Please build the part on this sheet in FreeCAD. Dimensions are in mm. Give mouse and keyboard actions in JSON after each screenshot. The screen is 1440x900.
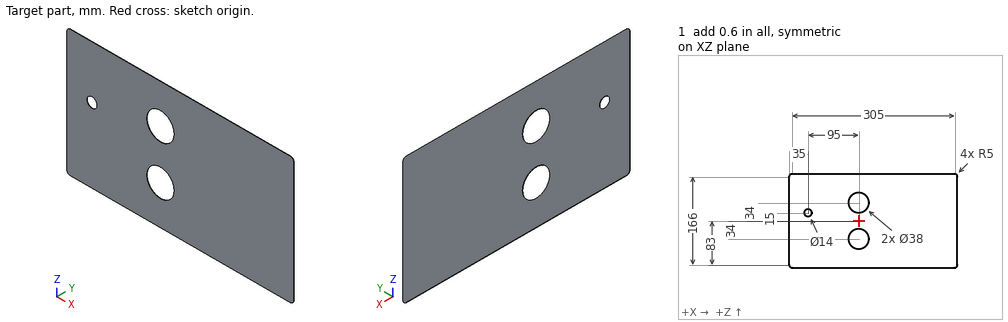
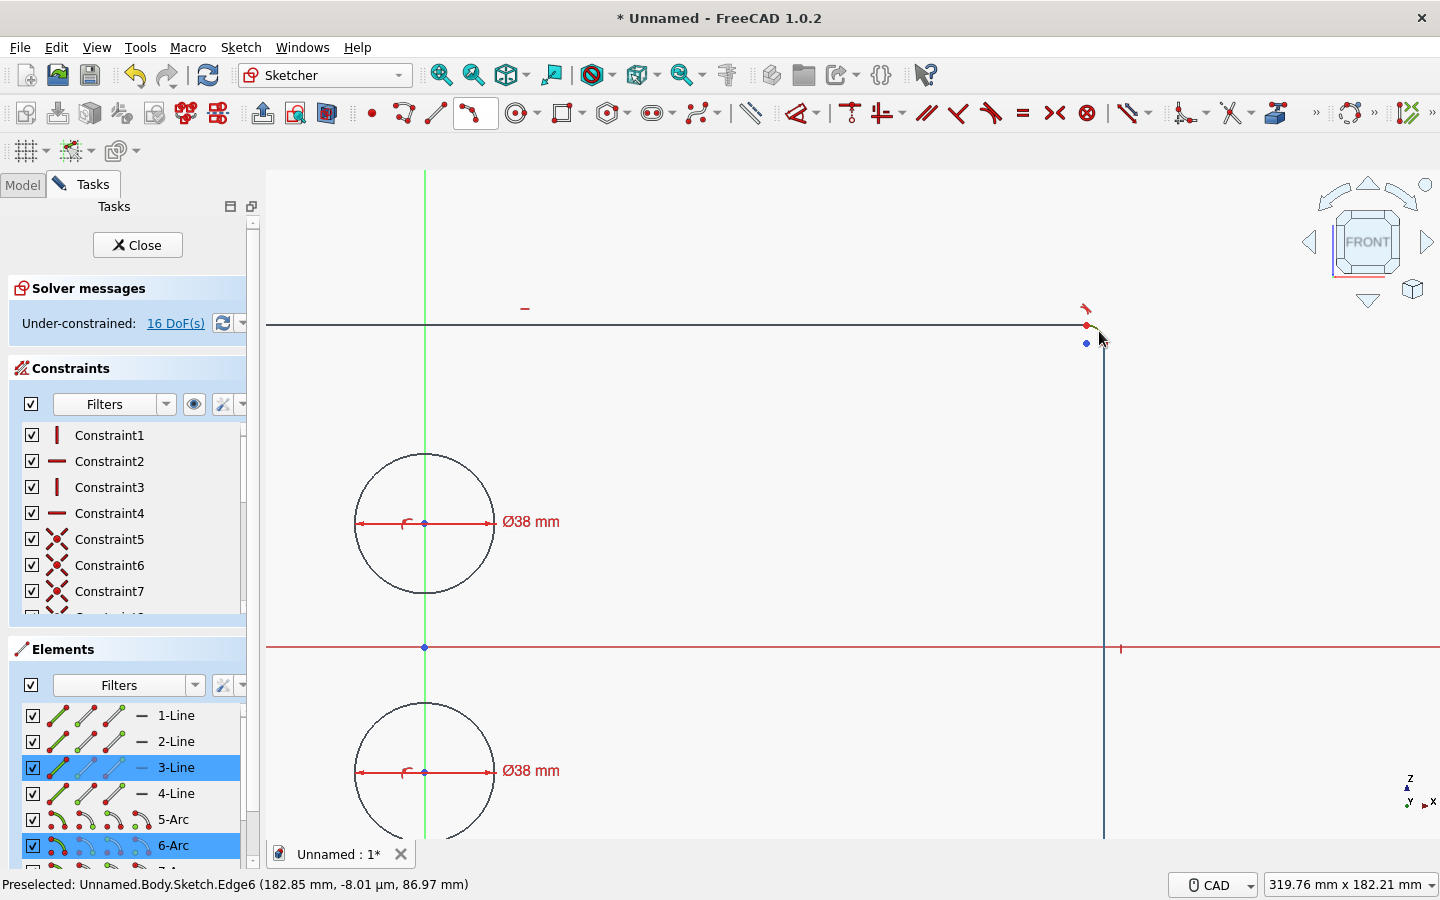
{"action": "left_click", "coordinate": [992, 114]}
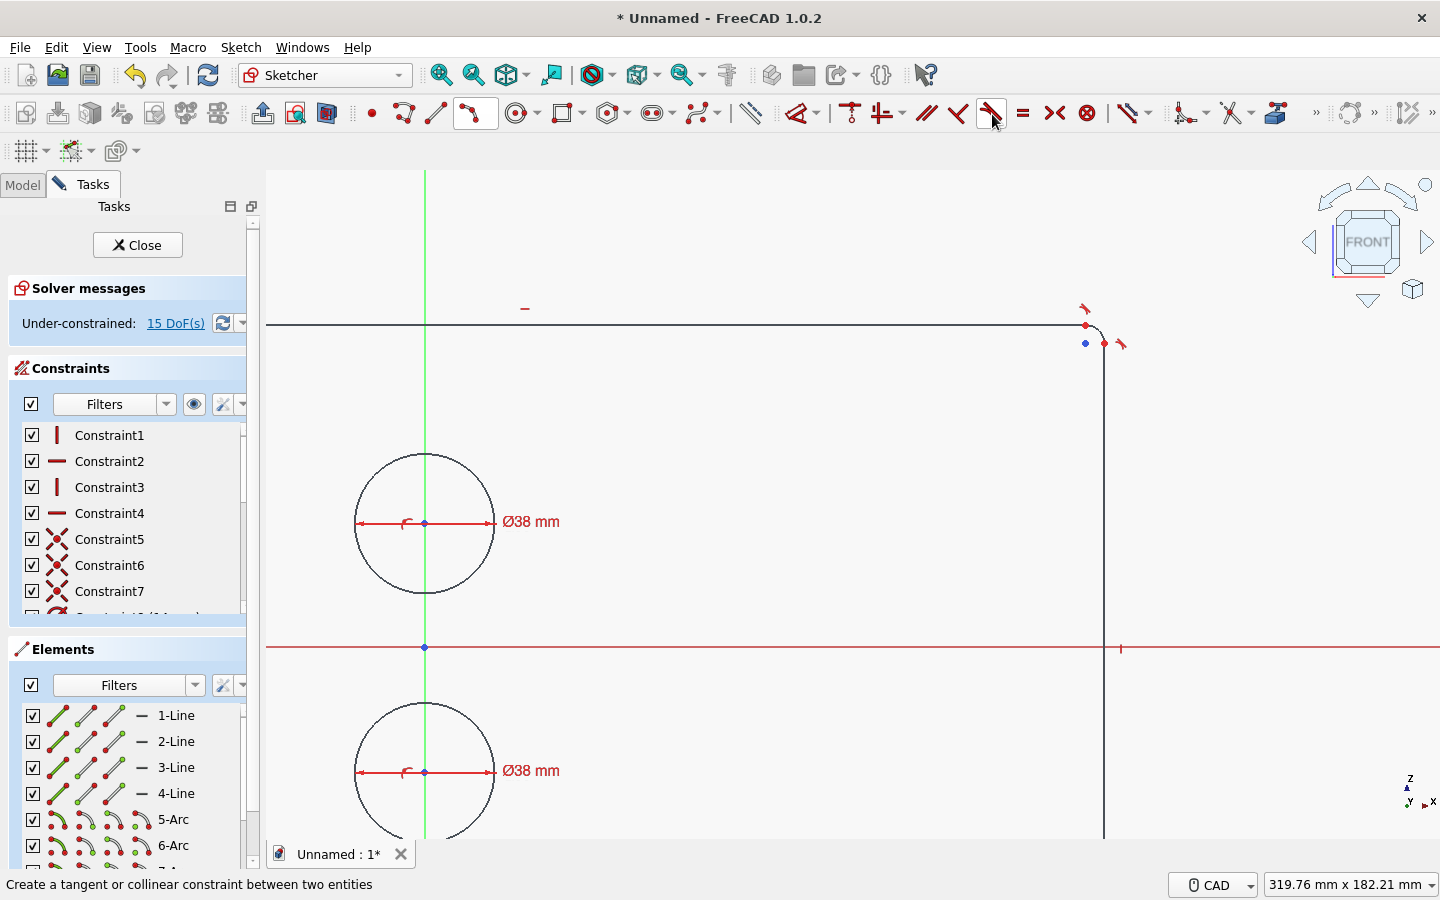
{"action": "left_click", "coordinate": [1104, 527]}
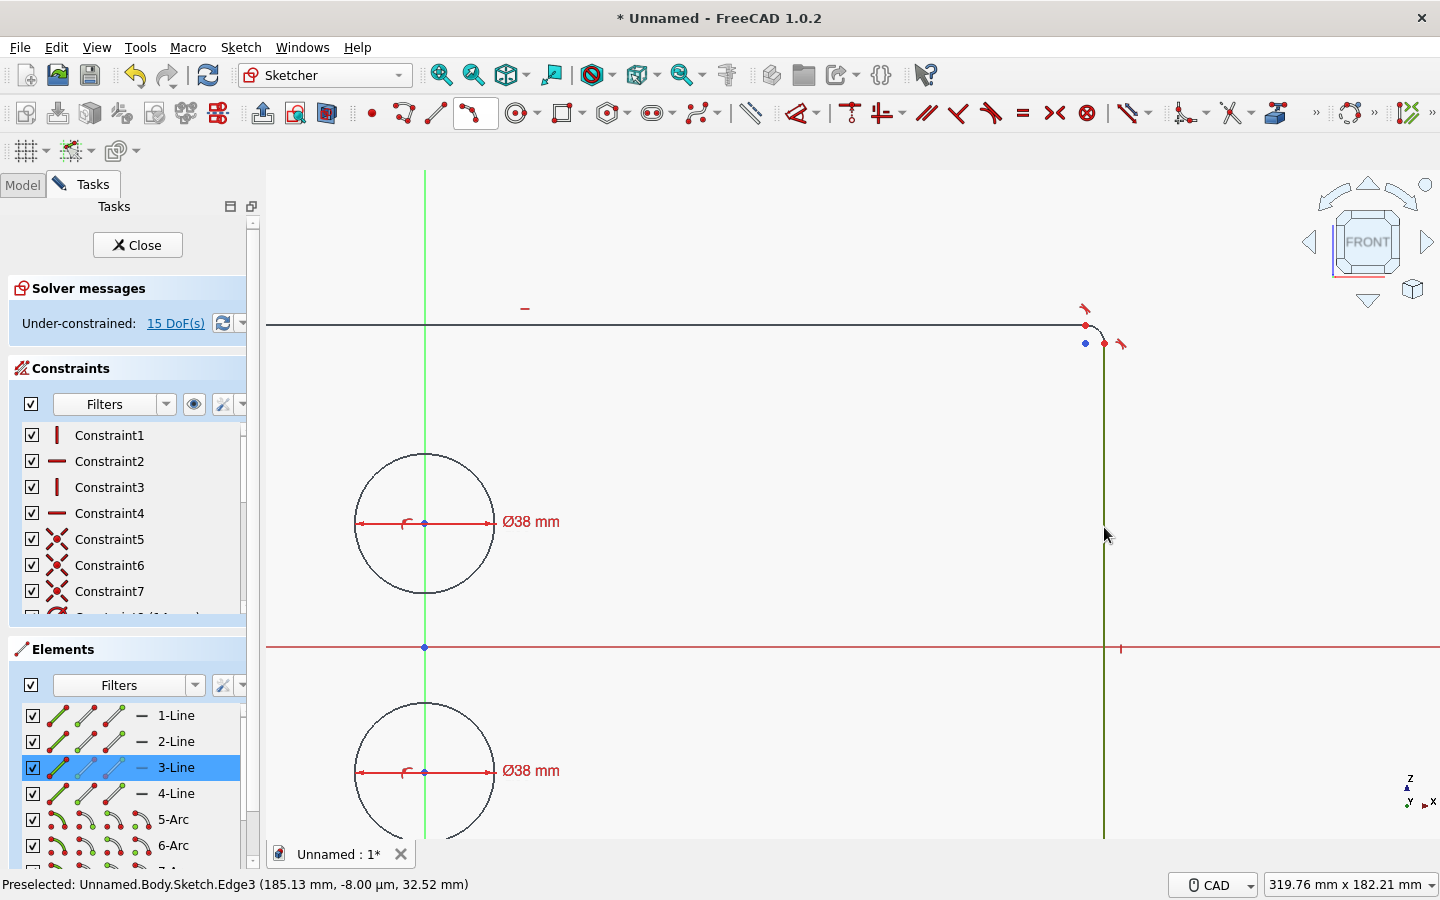
{"action": "scroll", "coordinate": [1099, 331], "scroll_direction": "down", "scroll_amount": 3}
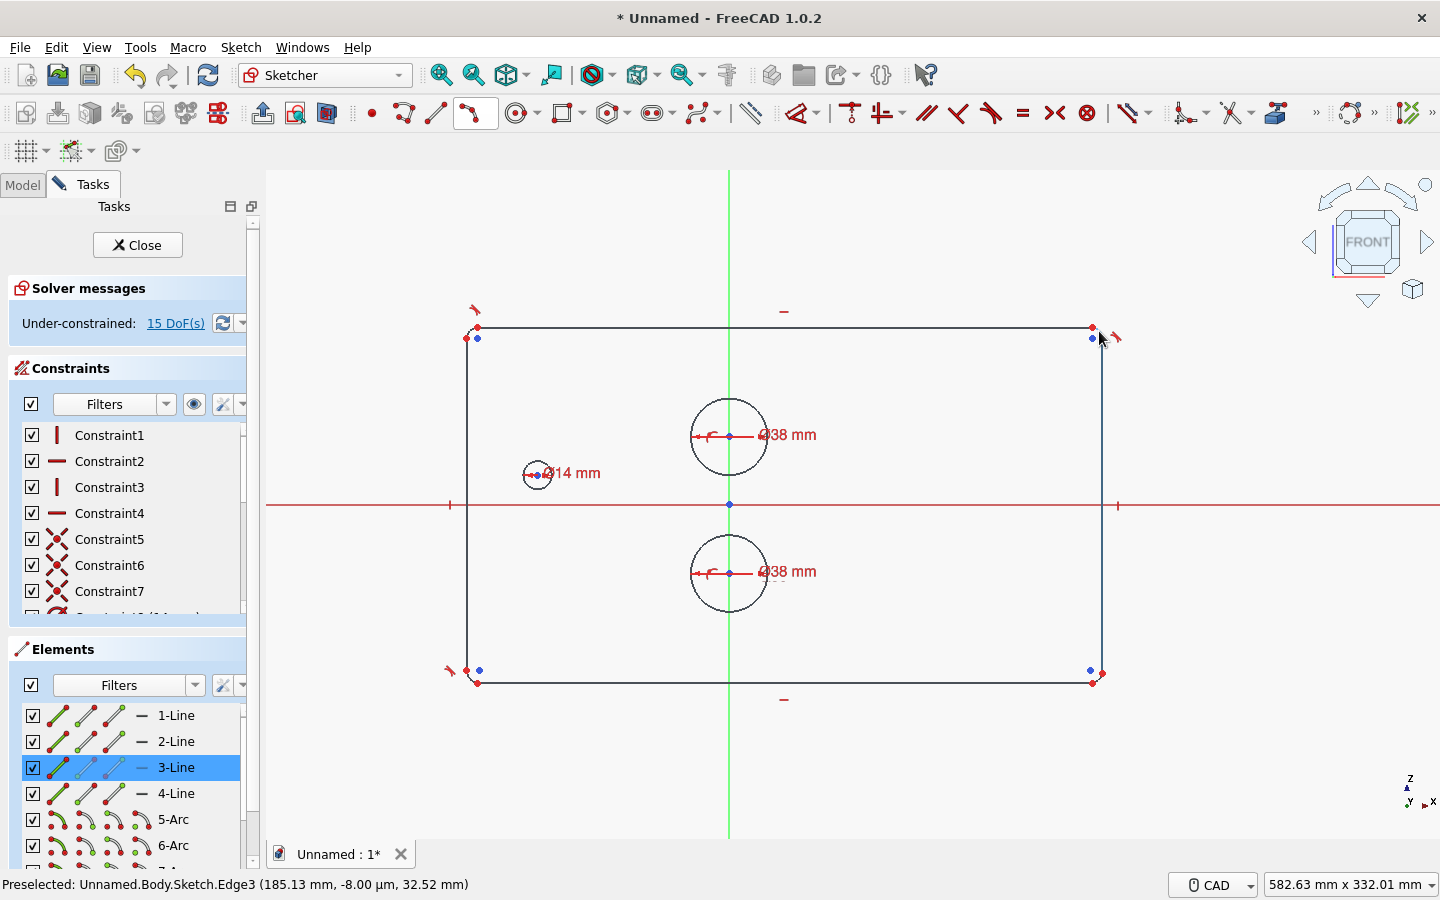
{"action": "scroll", "coordinate": [1099, 680], "scroll_direction": "up", "scroll_amount": 4}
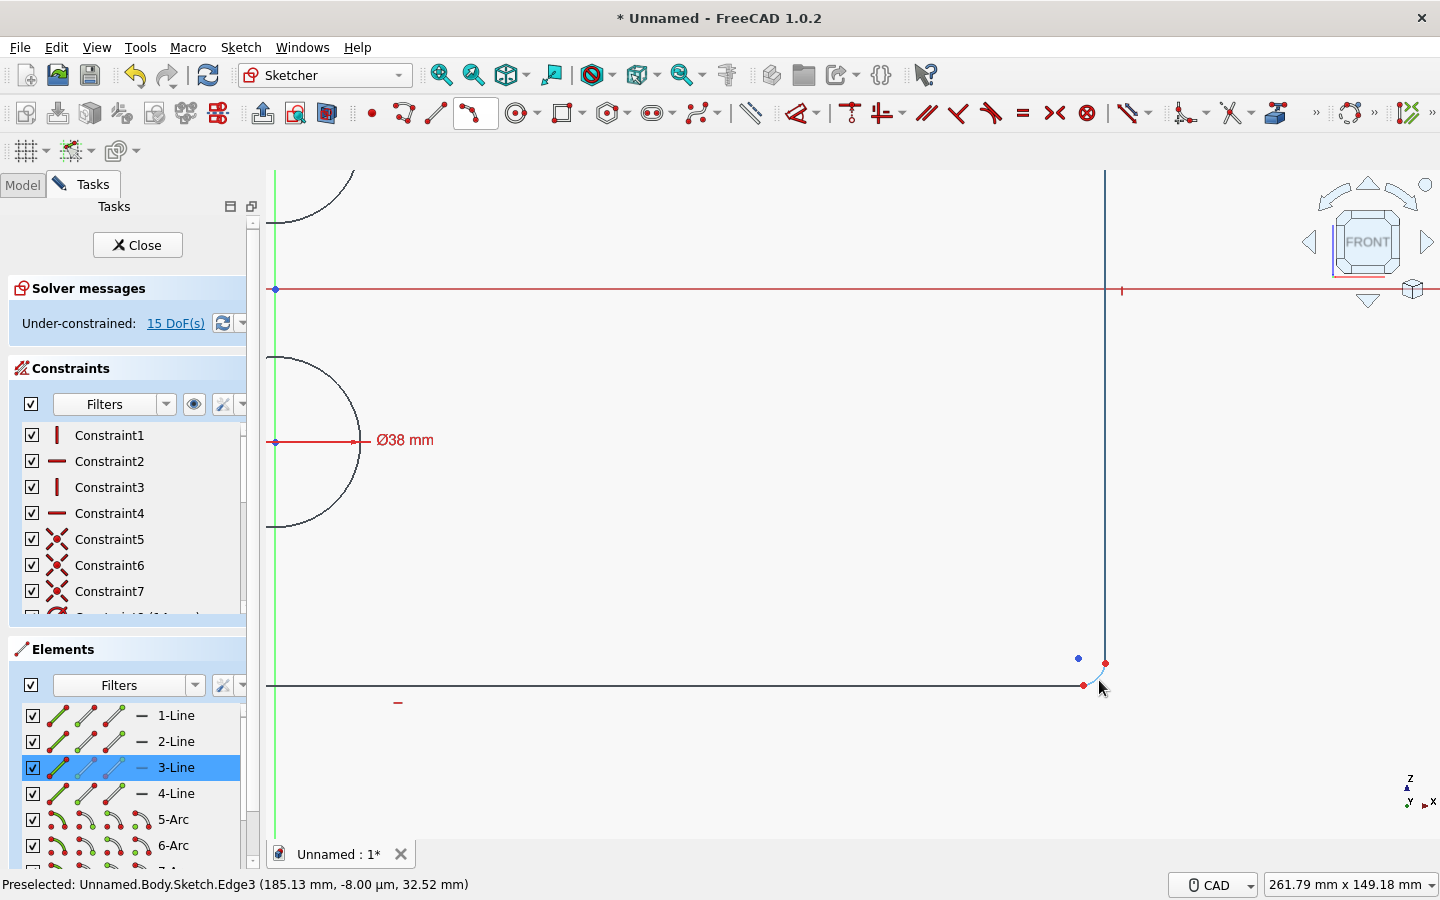
{"action": "left_click", "coordinate": [1098, 678]}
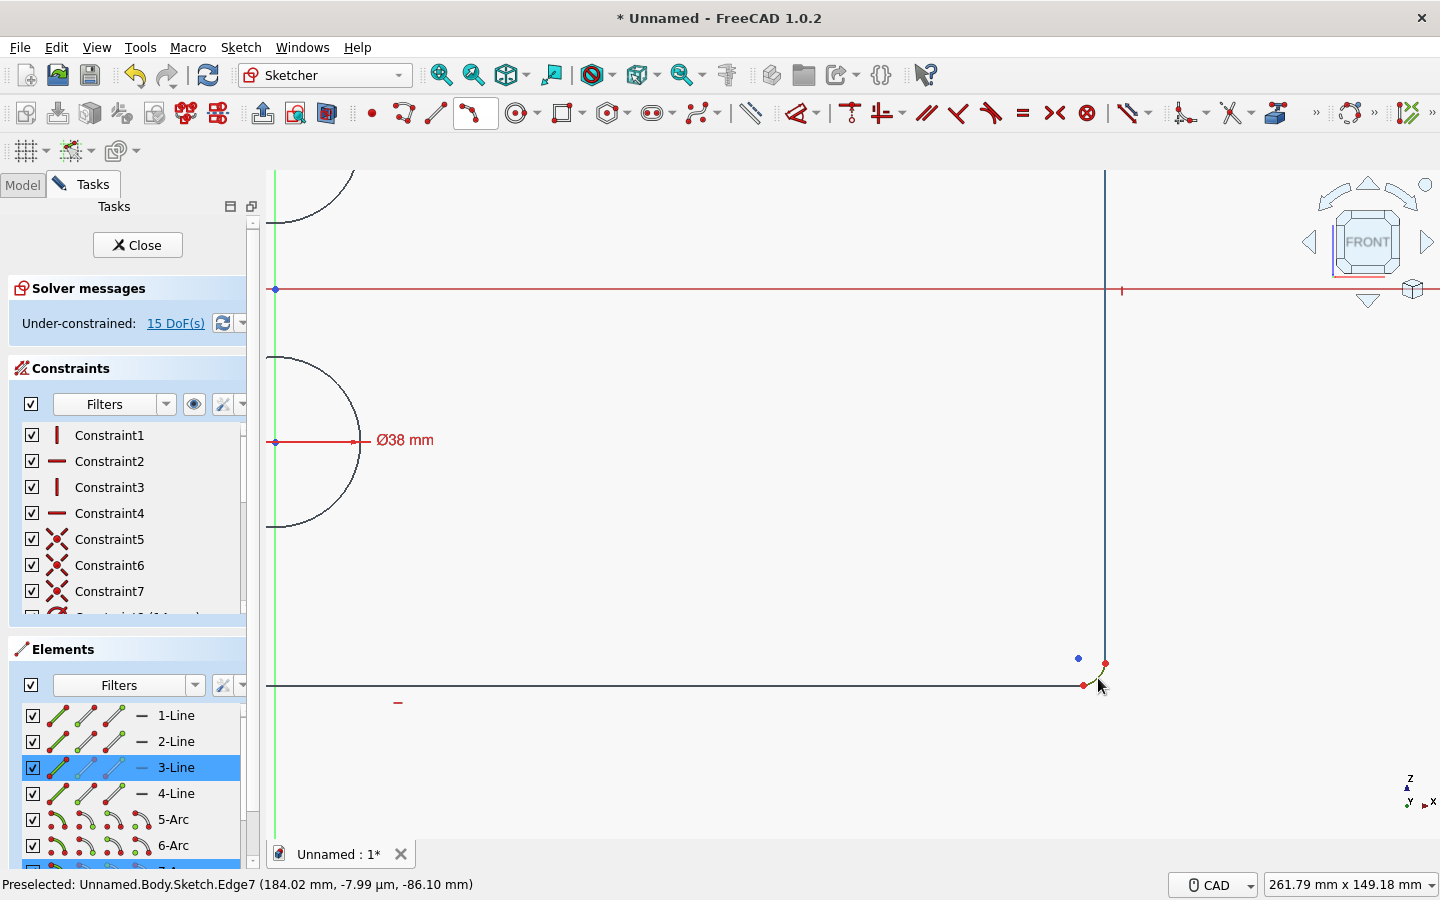
{"action": "left_click", "coordinate": [992, 114]}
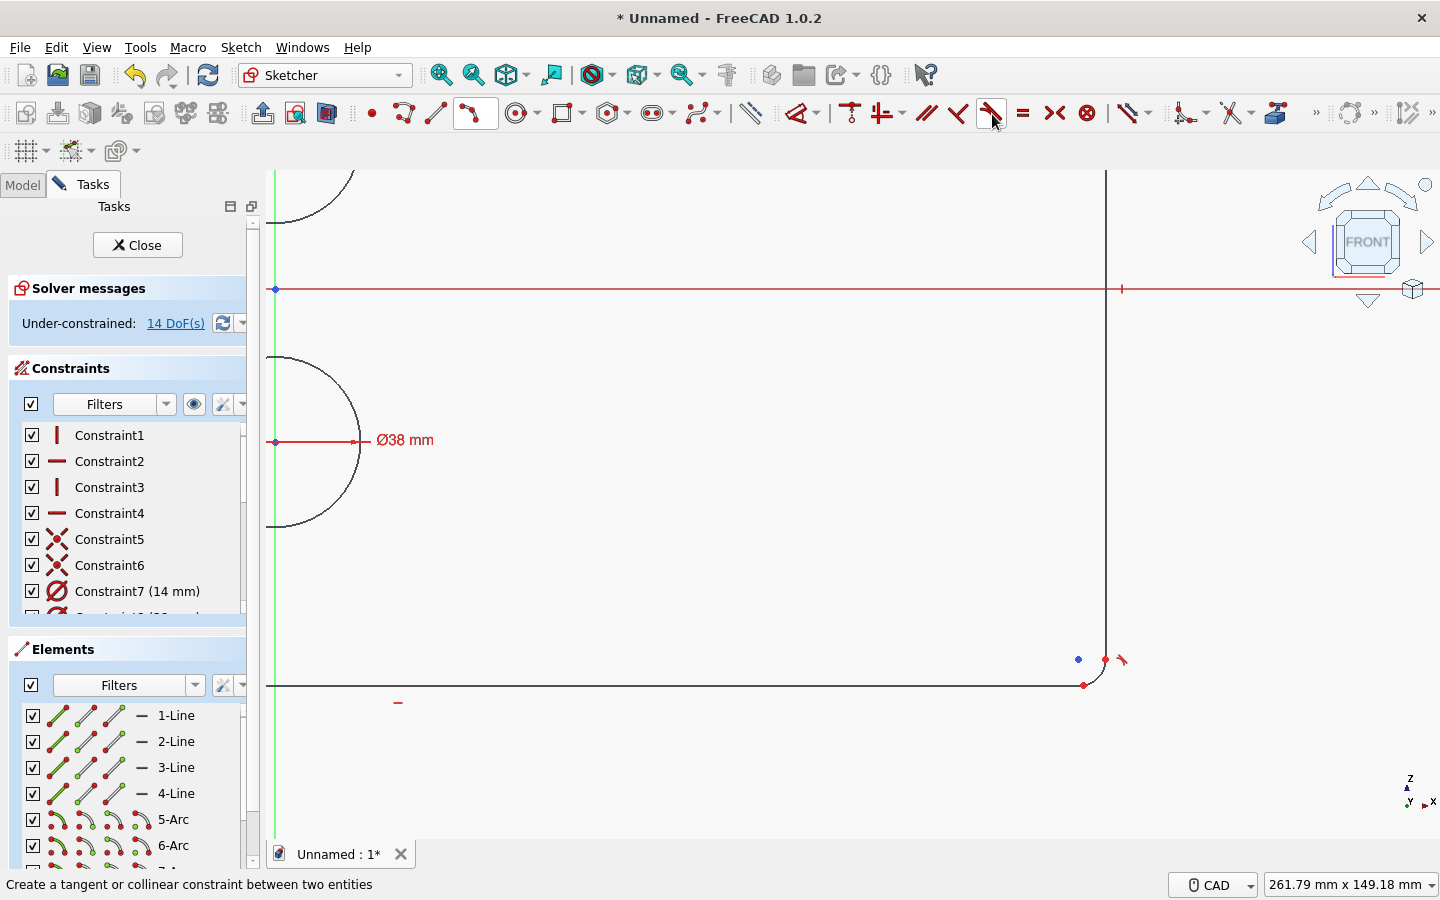
{"action": "left_click", "coordinate": [672, 686]}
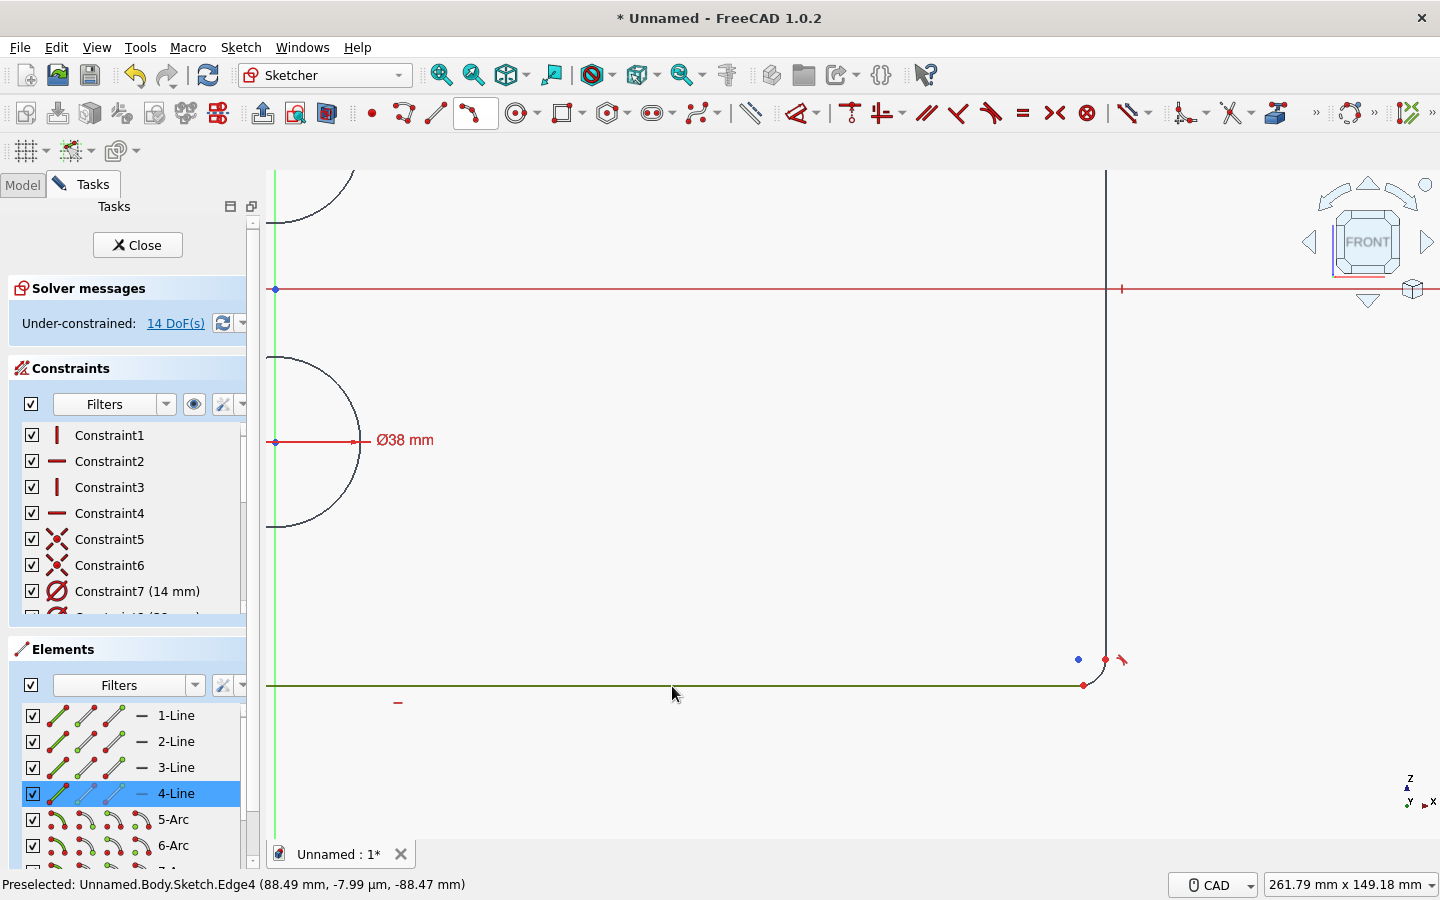
{"action": "left_click", "coordinate": [1094, 682]}